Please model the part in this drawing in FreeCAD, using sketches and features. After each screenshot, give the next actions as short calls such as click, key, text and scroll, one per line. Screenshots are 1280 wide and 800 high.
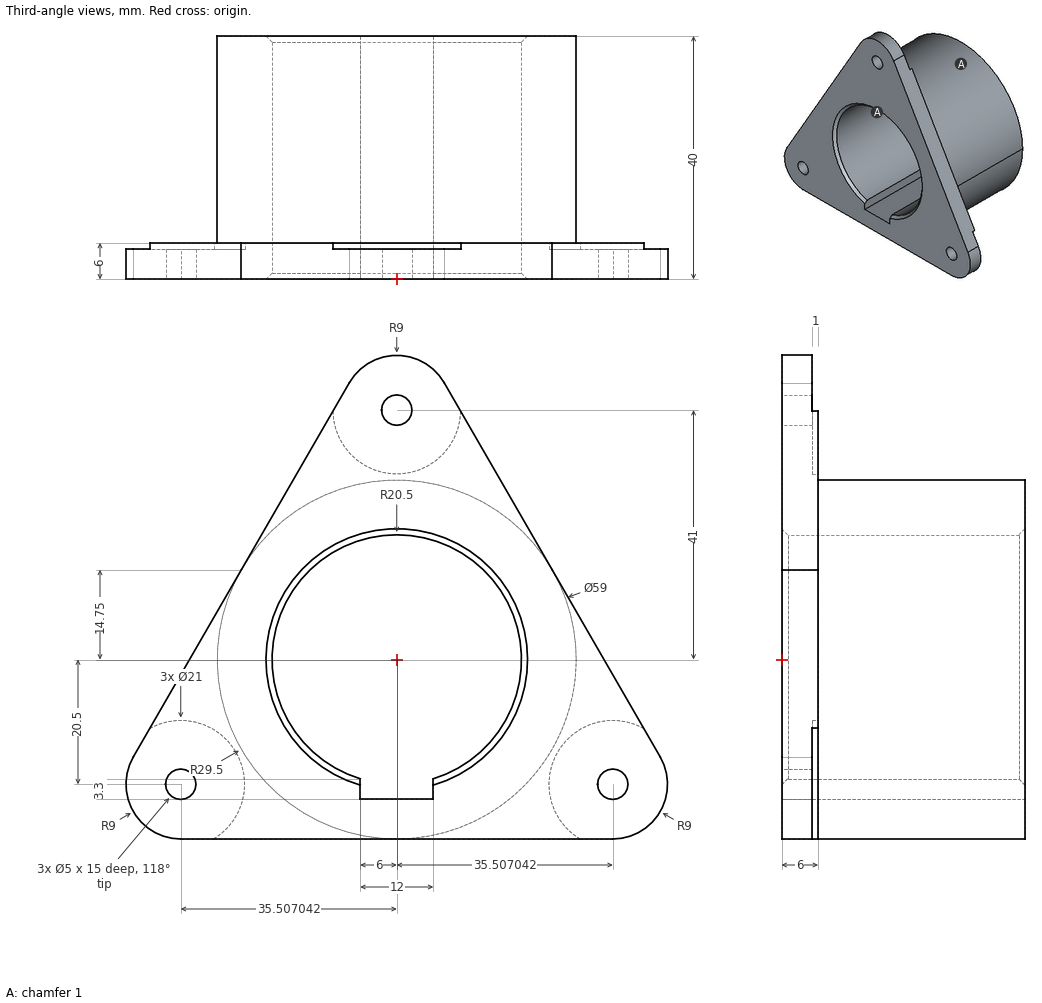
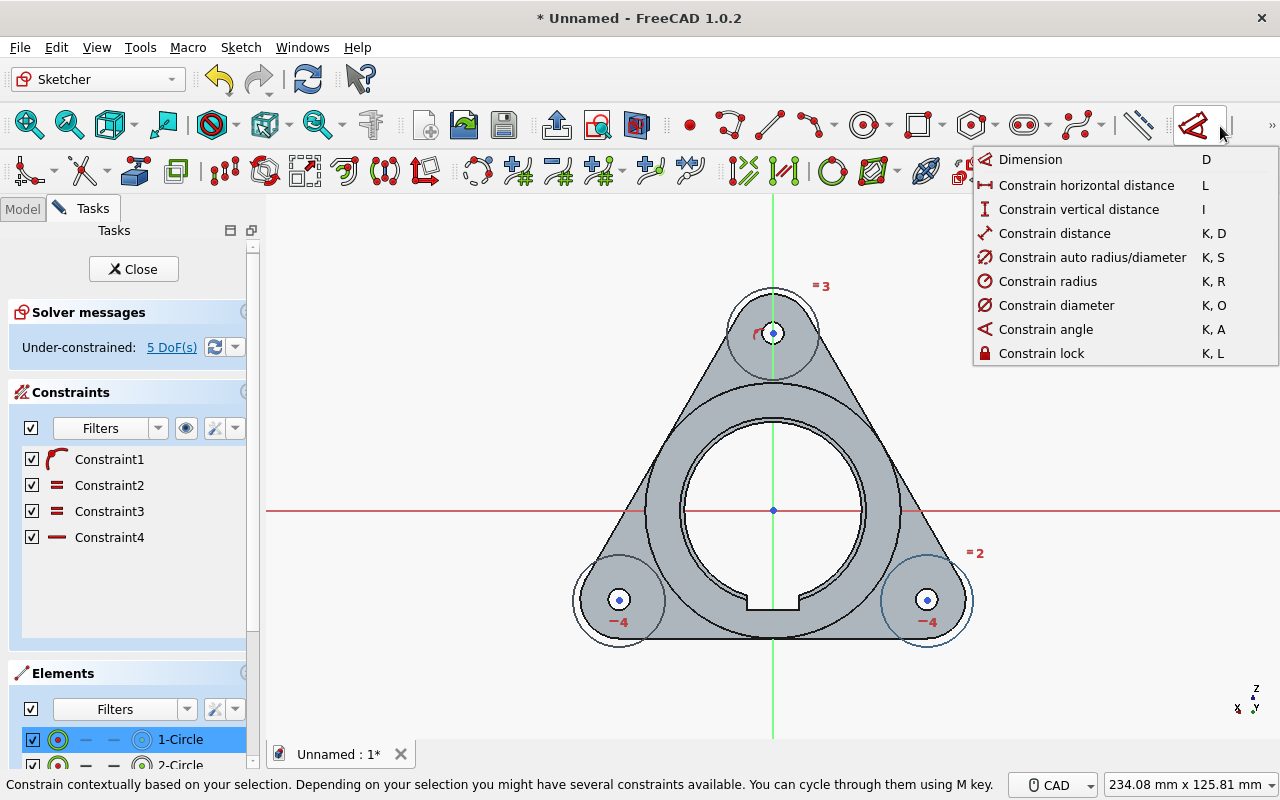
click(1126, 305)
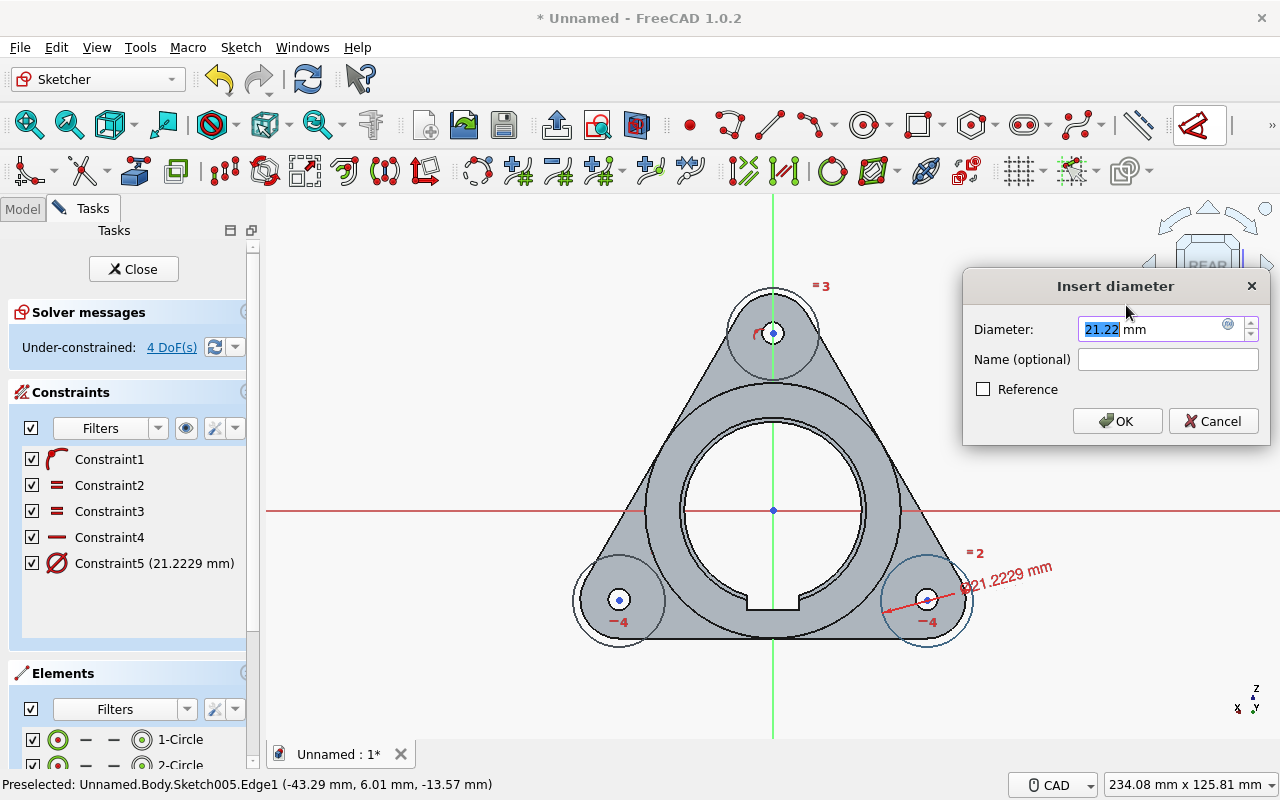
text(21)
key(Return)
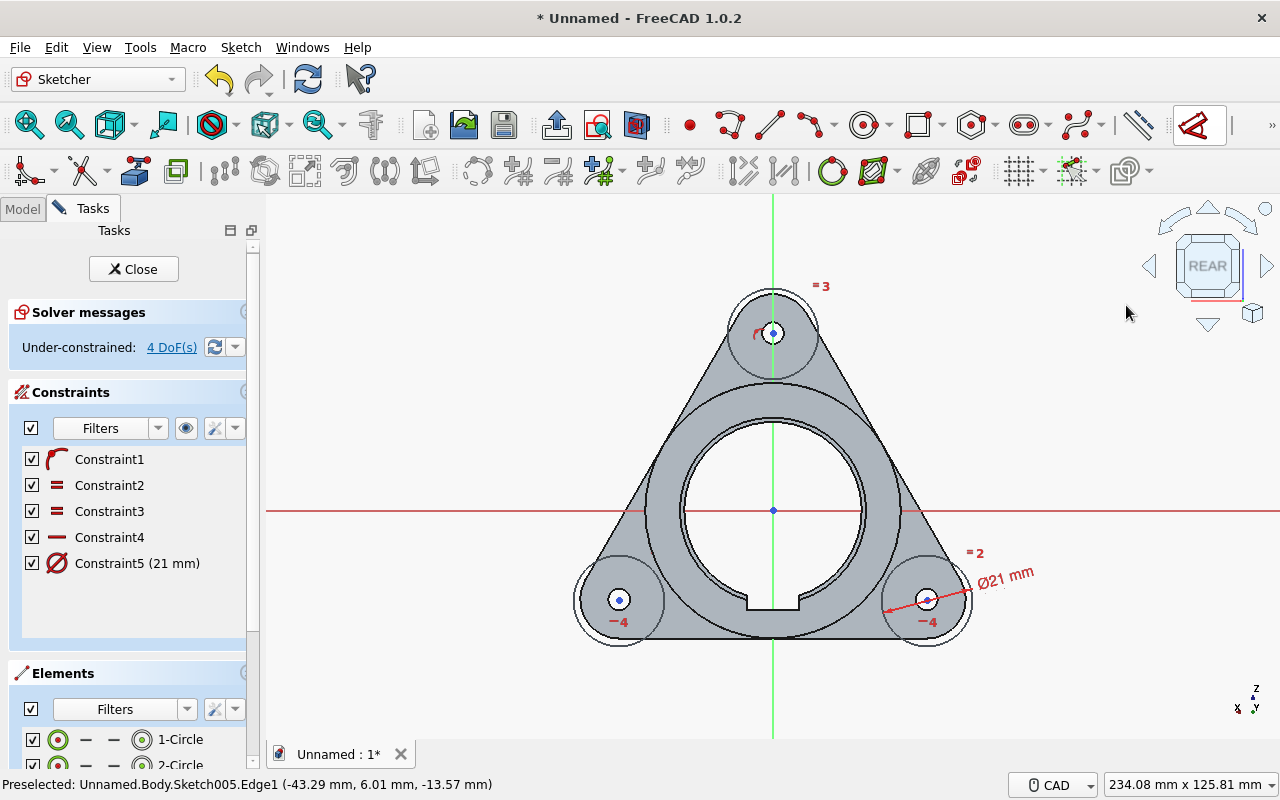
click(773, 334)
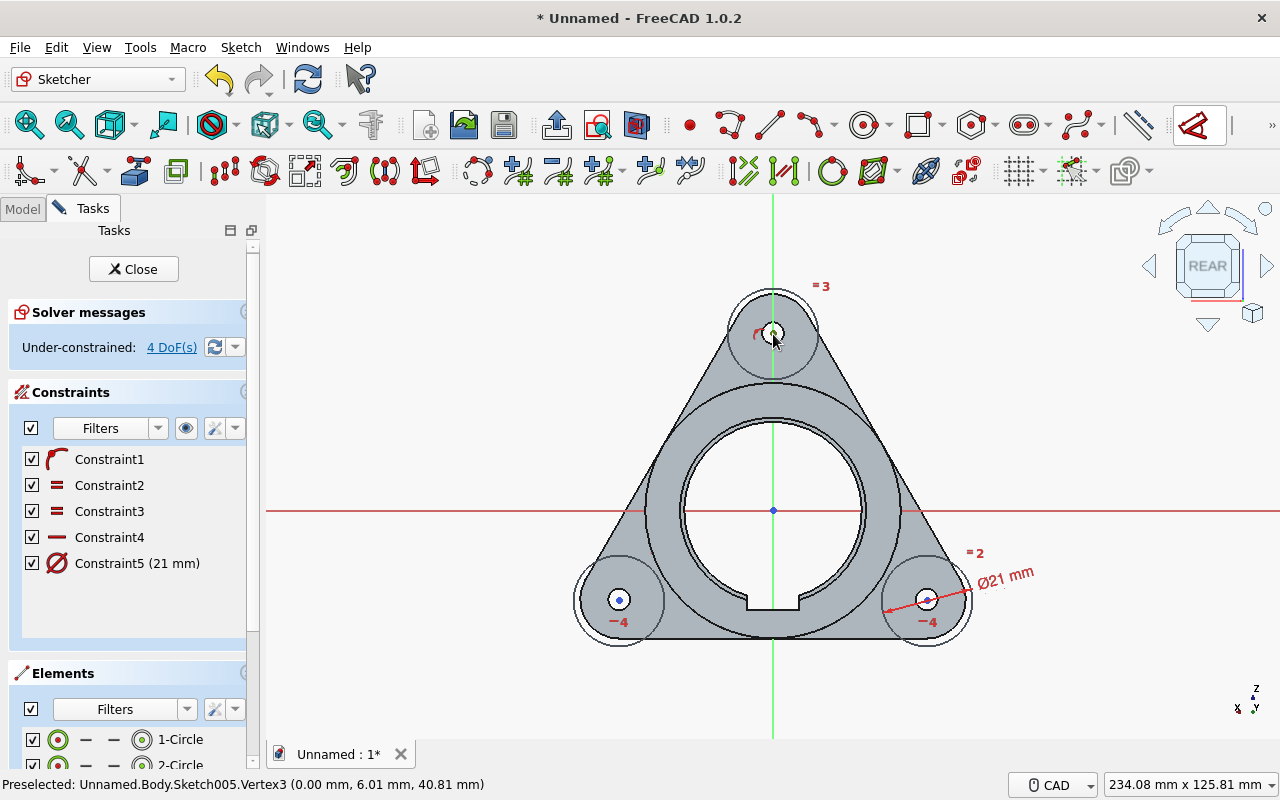
key(i)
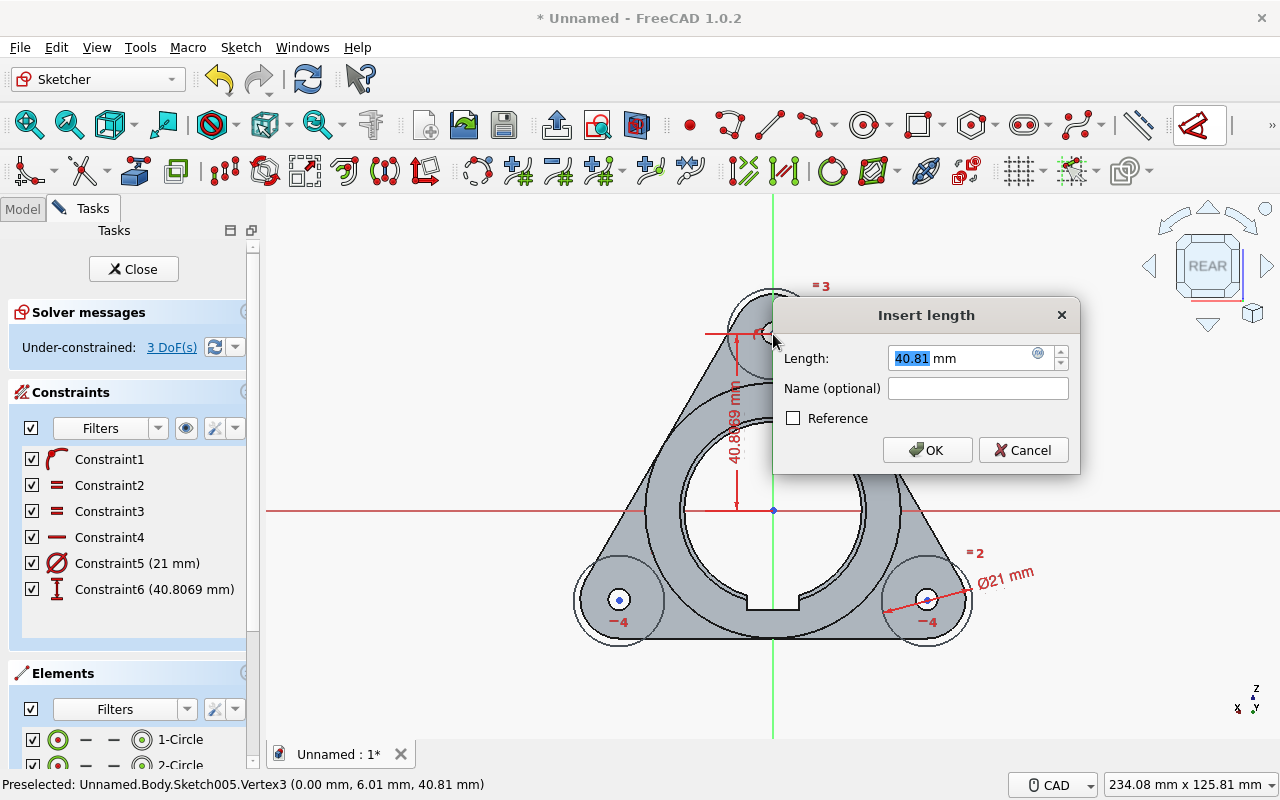
text(41)
key(Return)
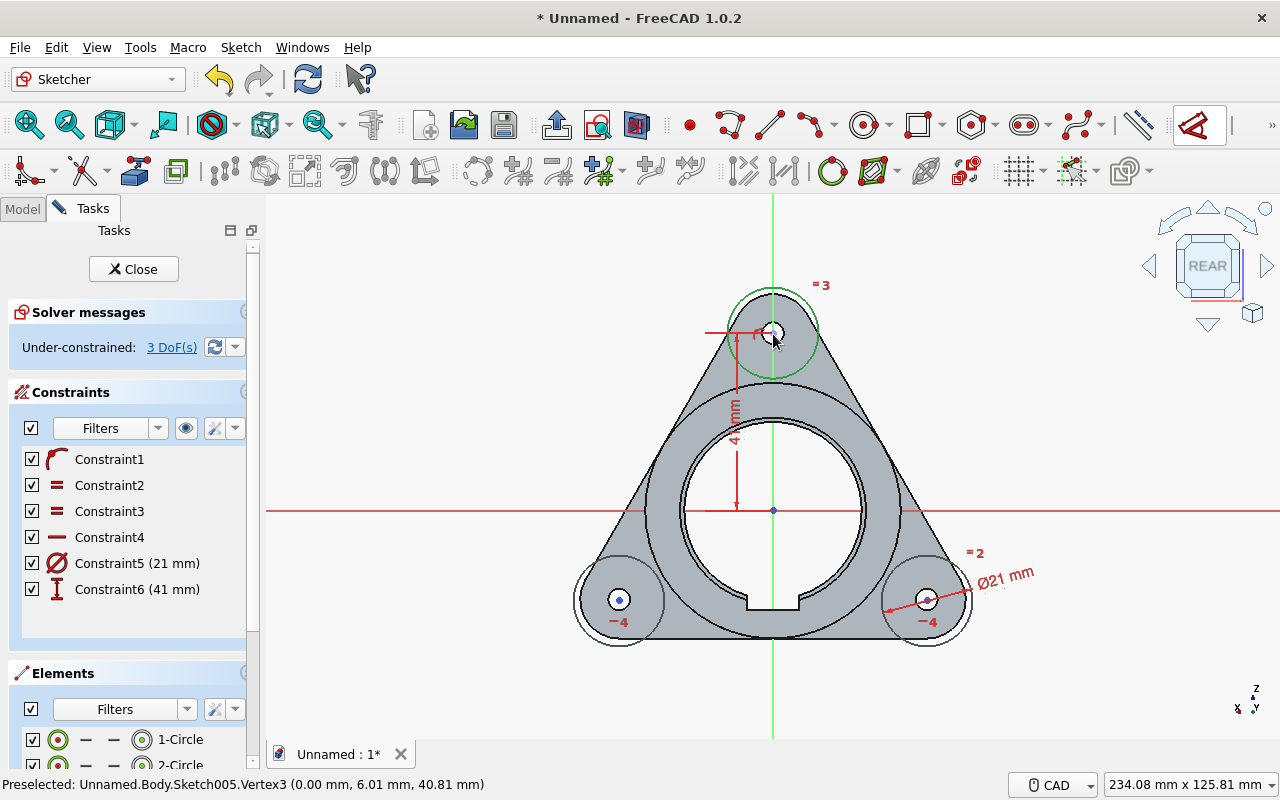
click(927, 601)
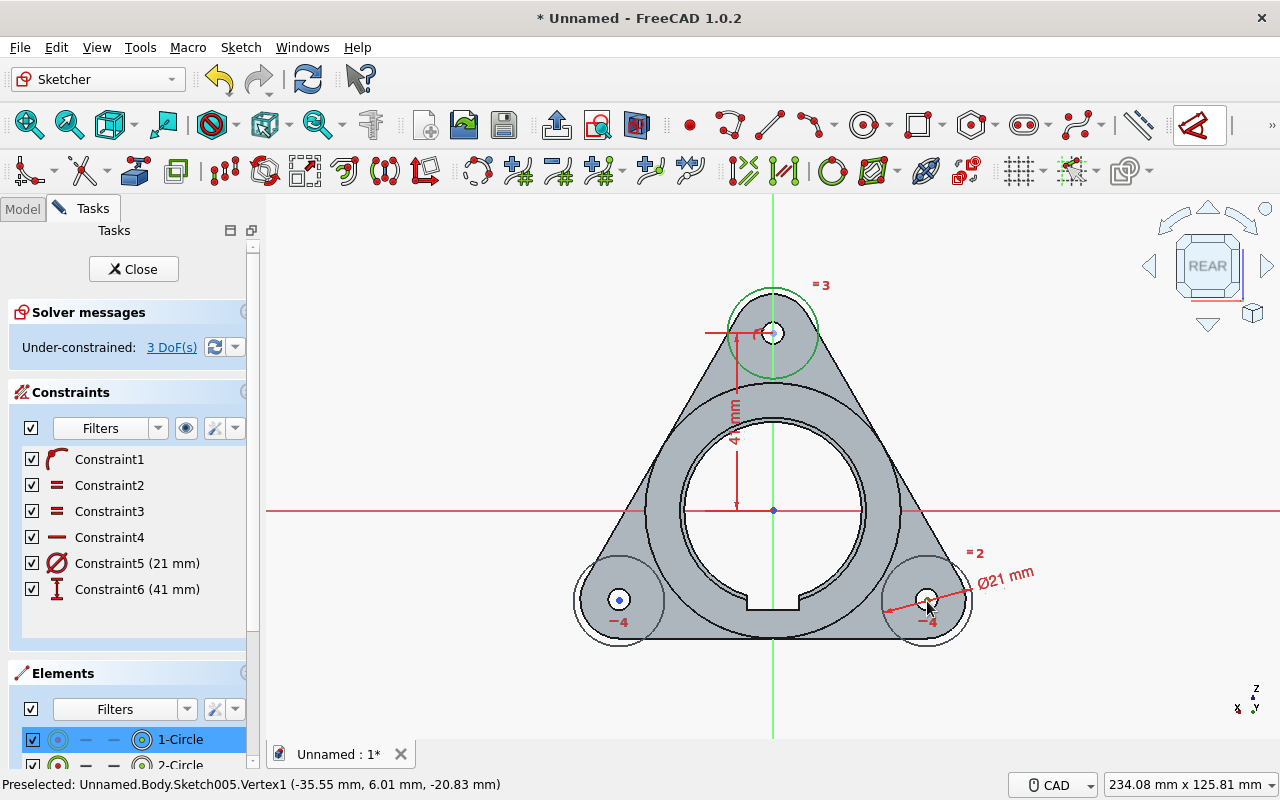
click(1220, 126)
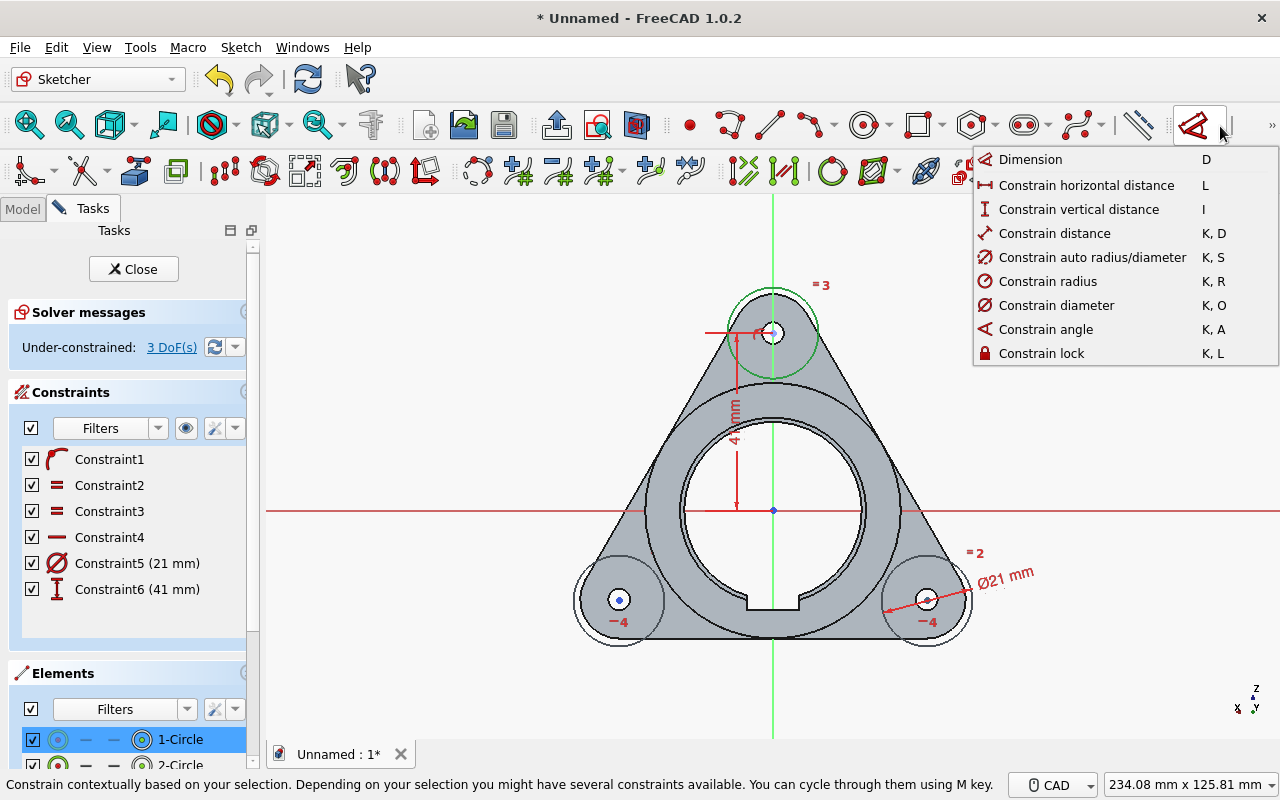
click(1126, 209)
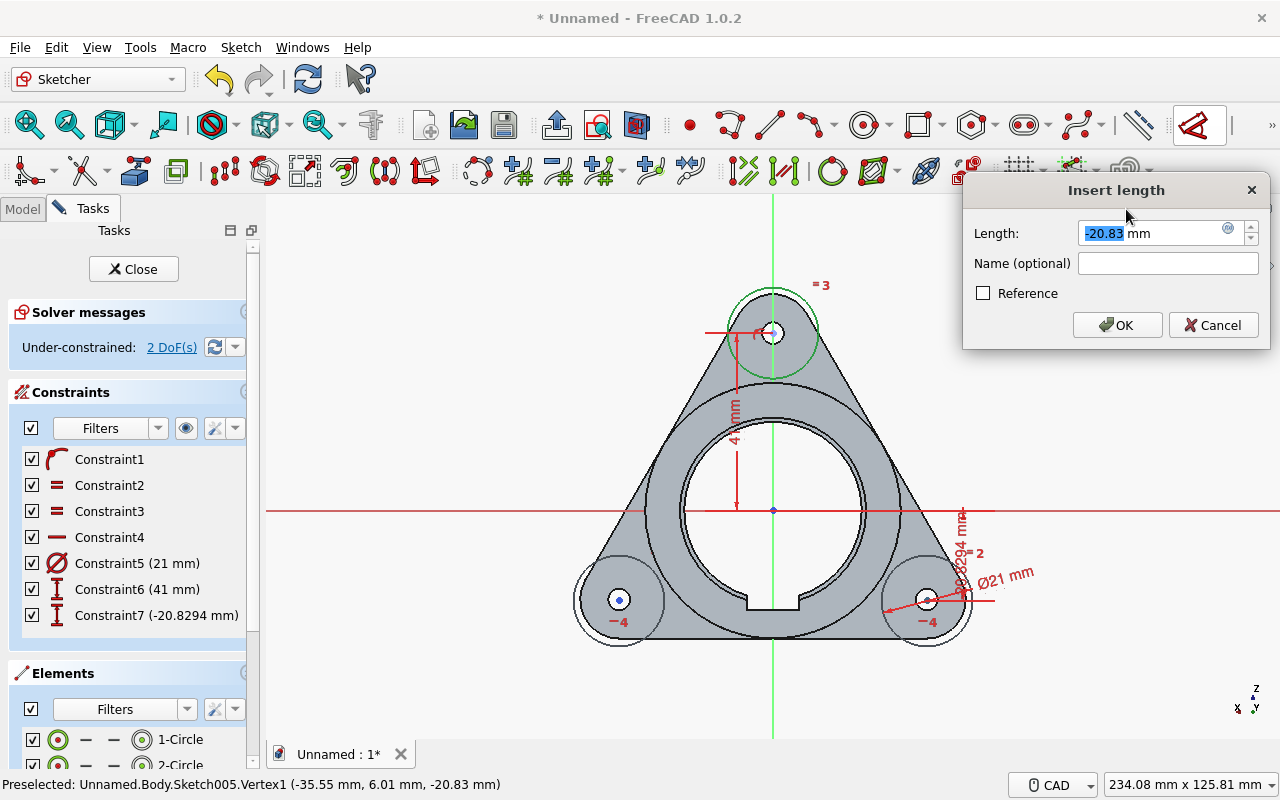
text(-20.5)
key(Return)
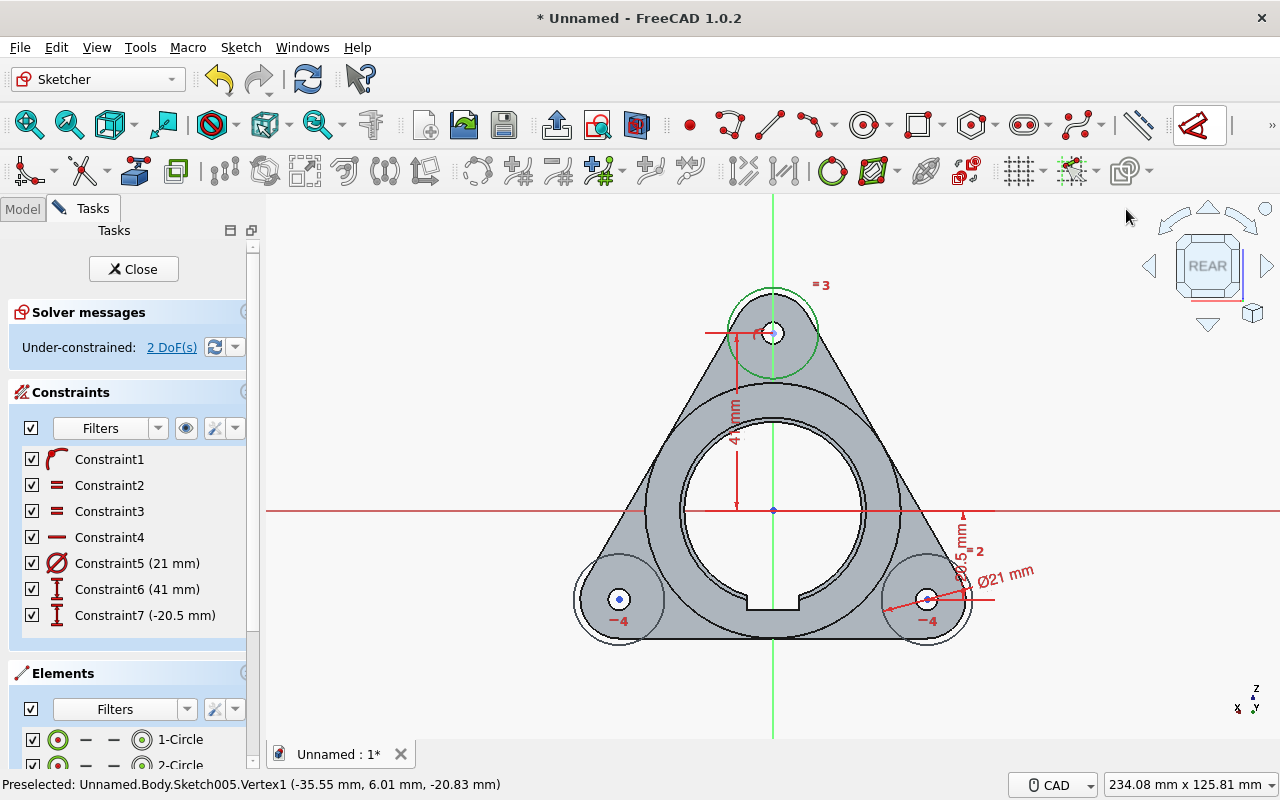
click(927, 600)